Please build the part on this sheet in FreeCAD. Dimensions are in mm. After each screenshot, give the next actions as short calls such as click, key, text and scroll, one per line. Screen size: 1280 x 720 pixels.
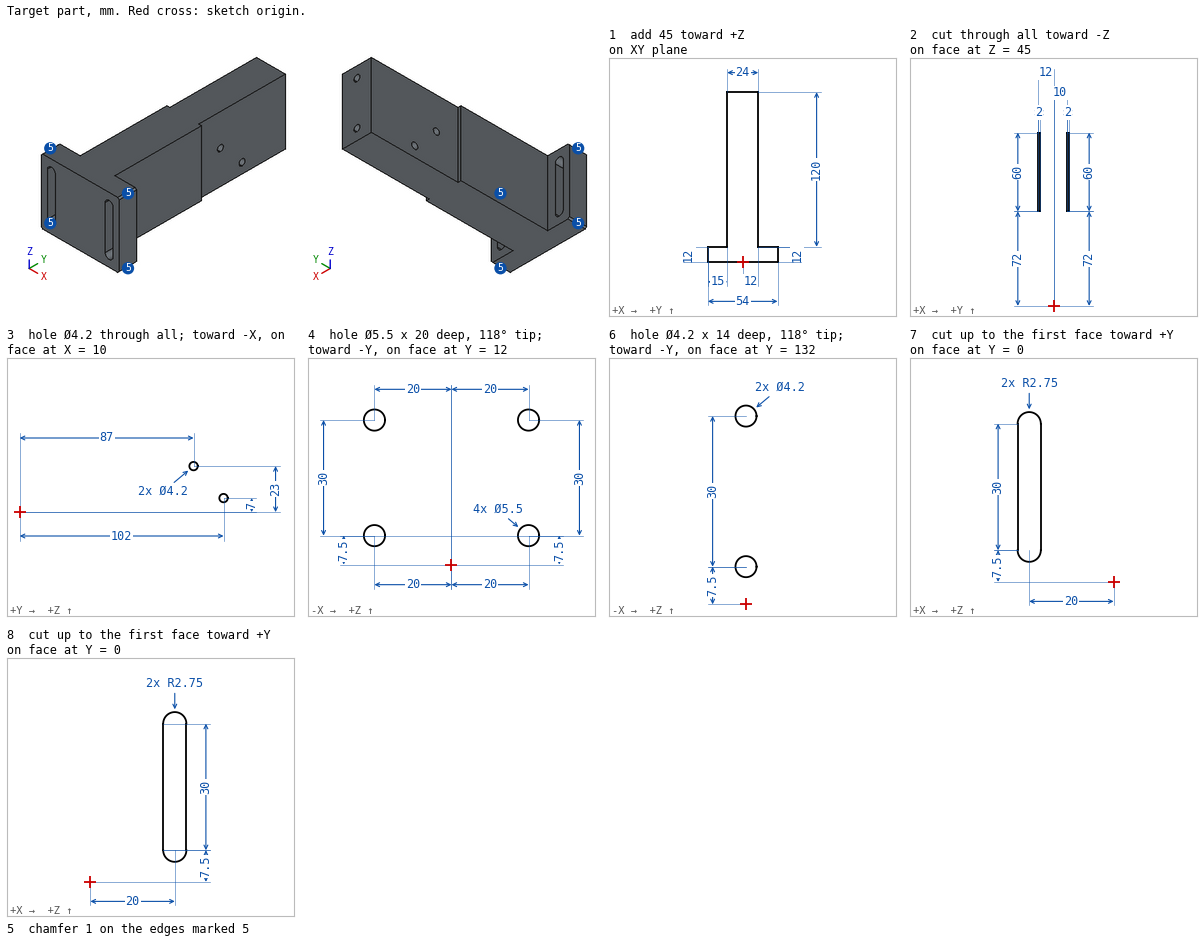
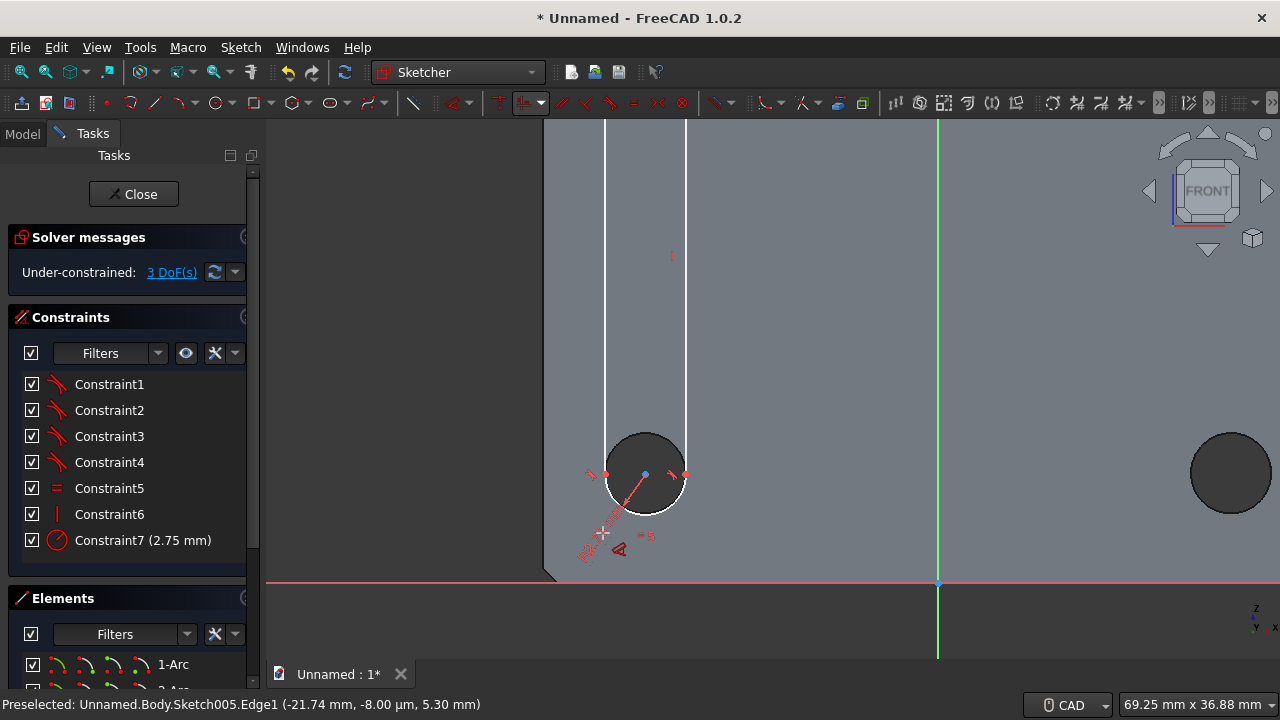
click(605, 343)
click(571, 311)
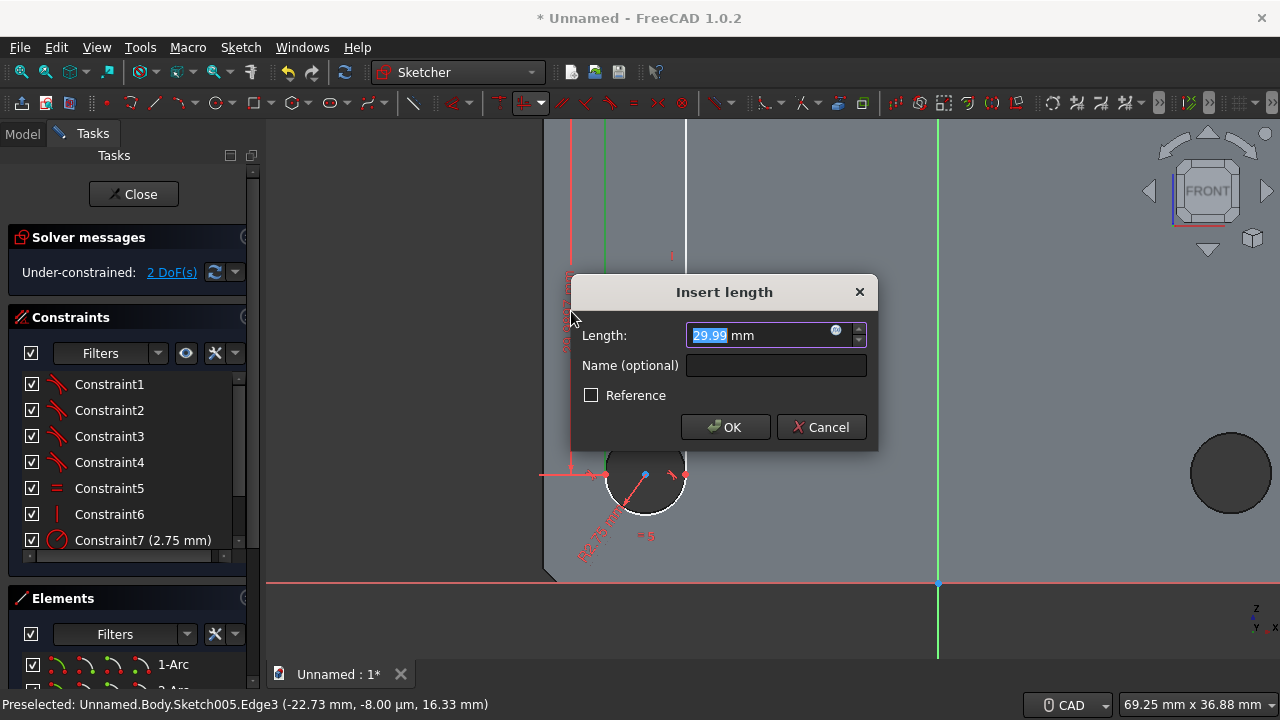
text(30)
key(Return)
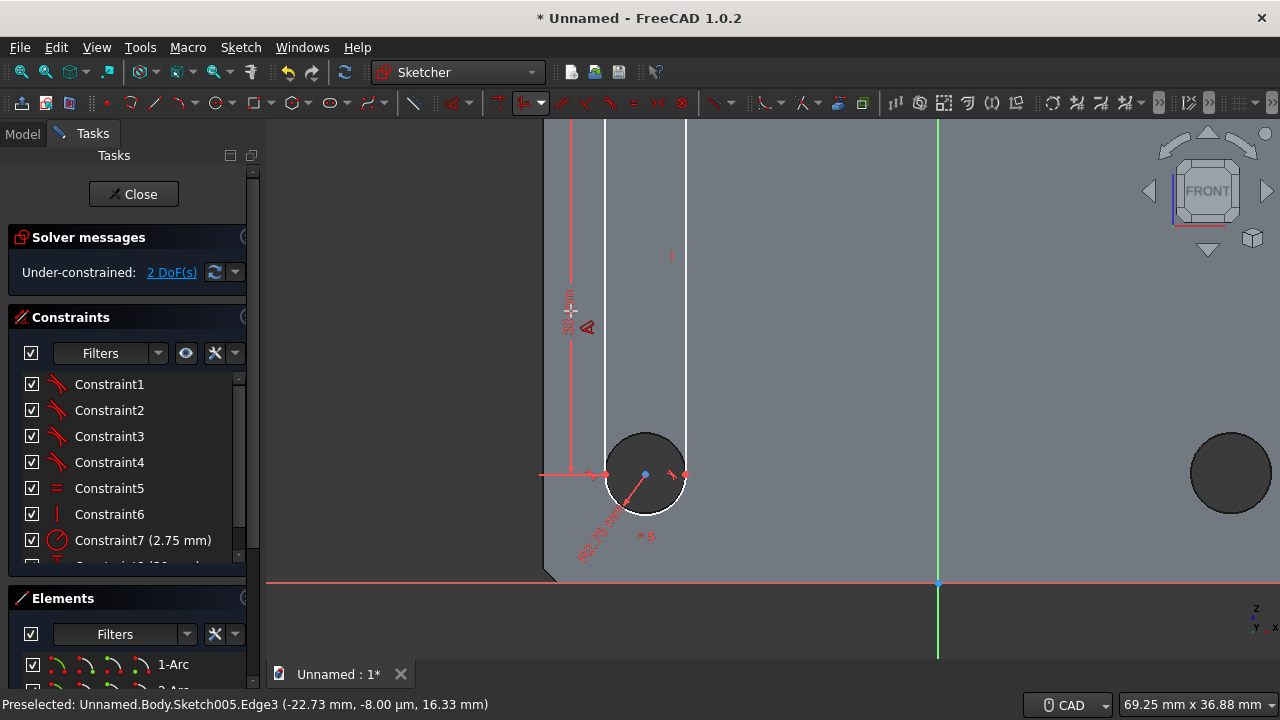
click(646, 475)
click(792, 617)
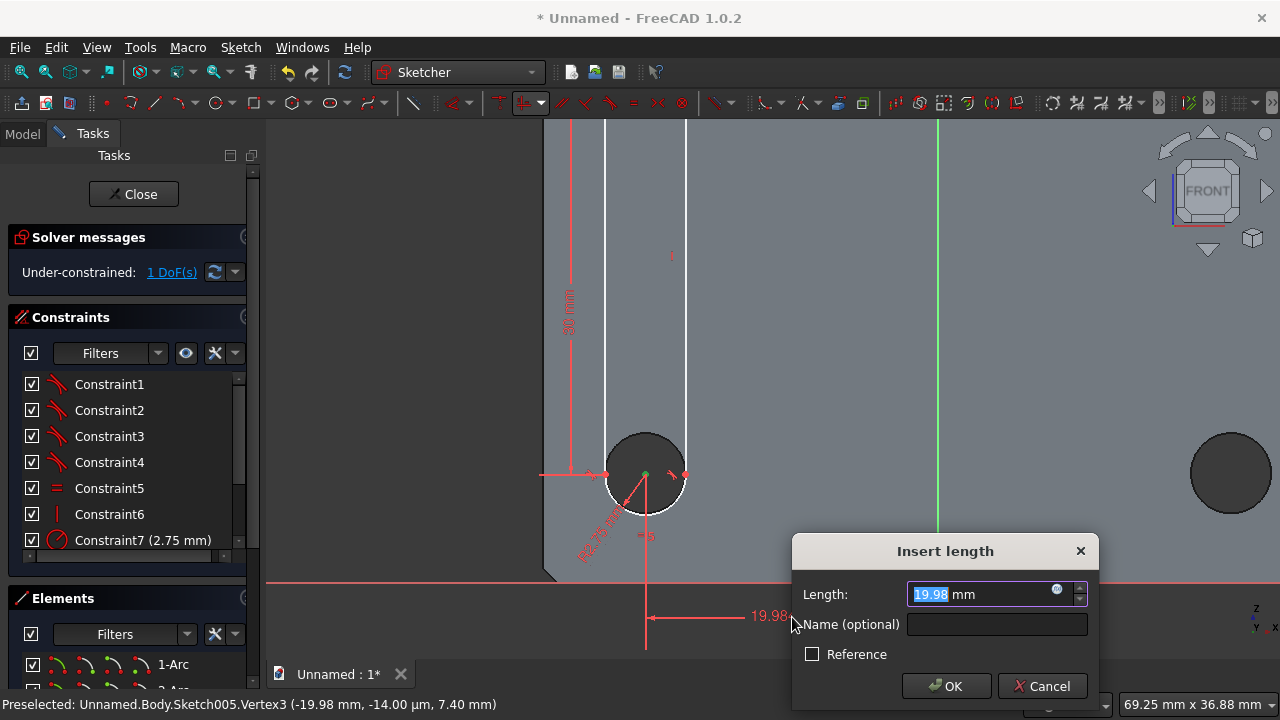
text(20)
key(Return)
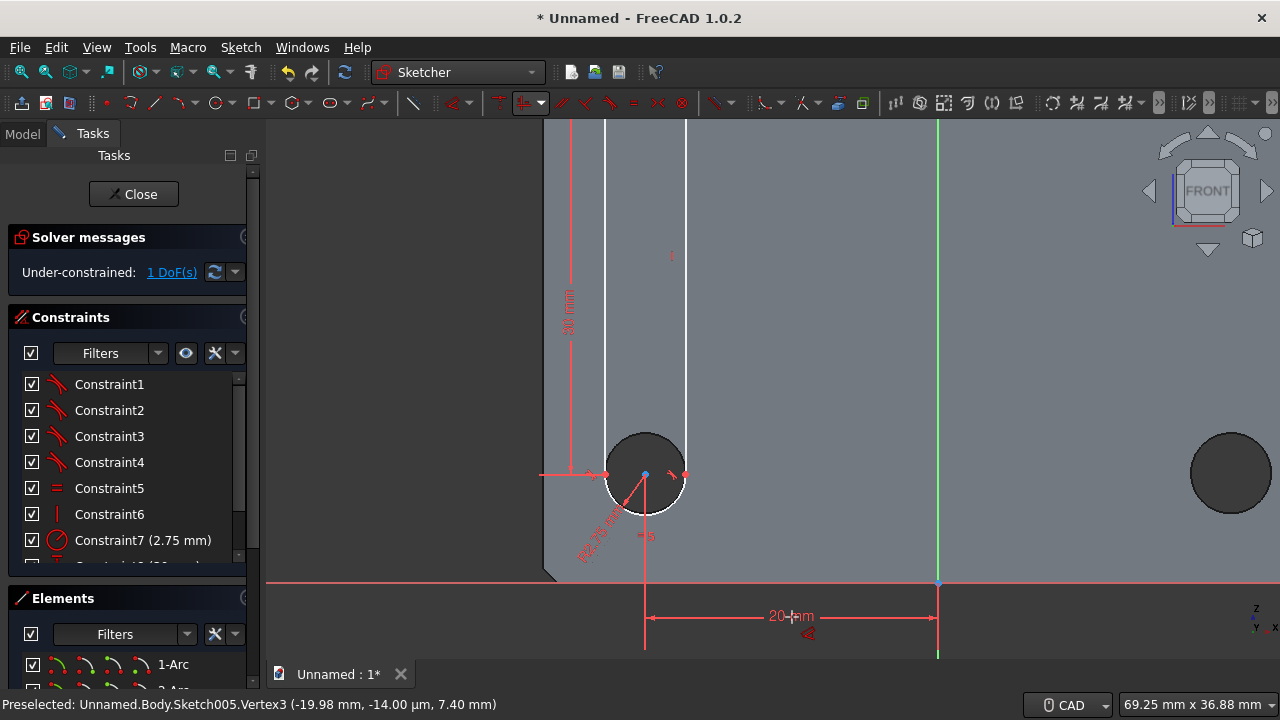
click(605, 475)
click(972, 529)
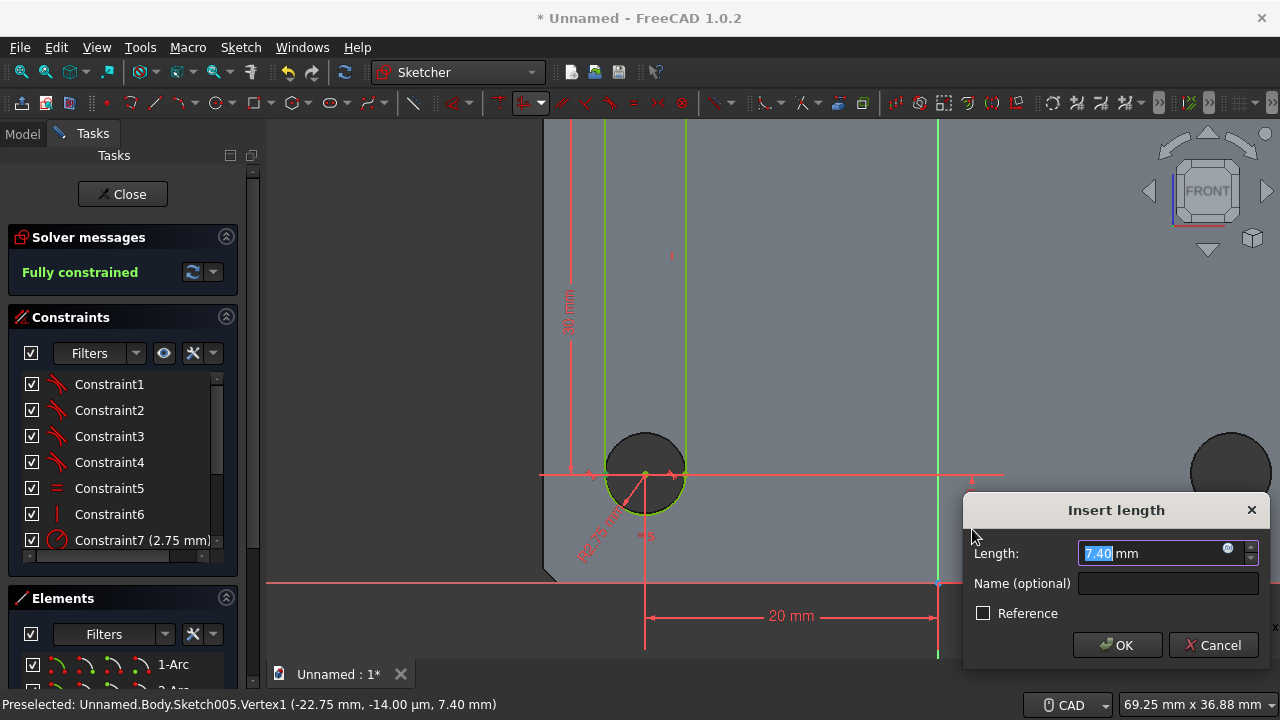
text(7.5)
key(Return)
key(Escape)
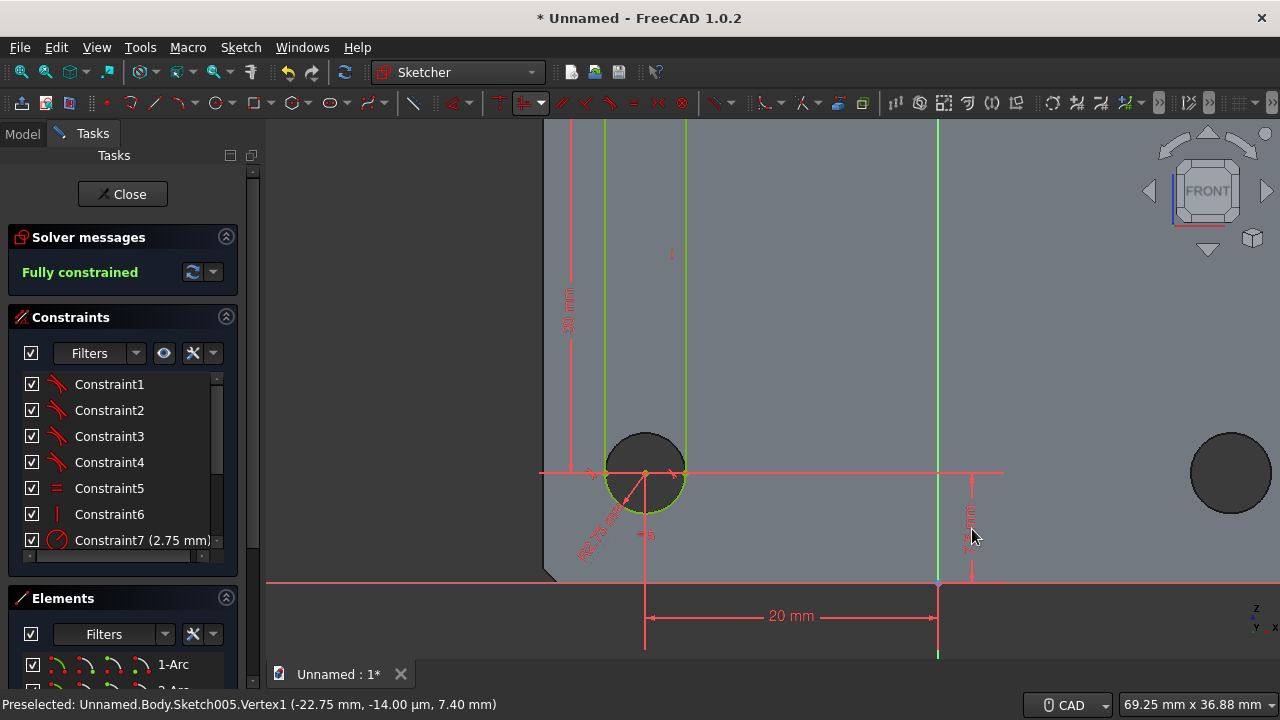
click(123, 194)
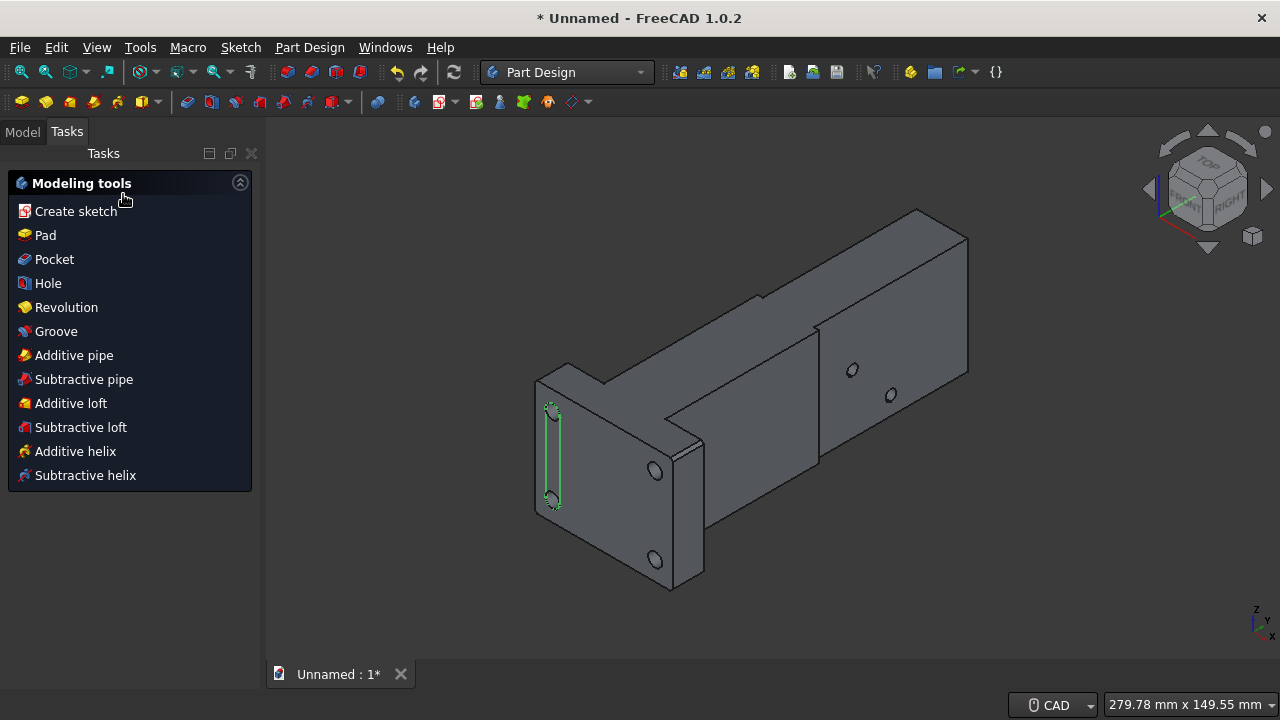
click(188, 102)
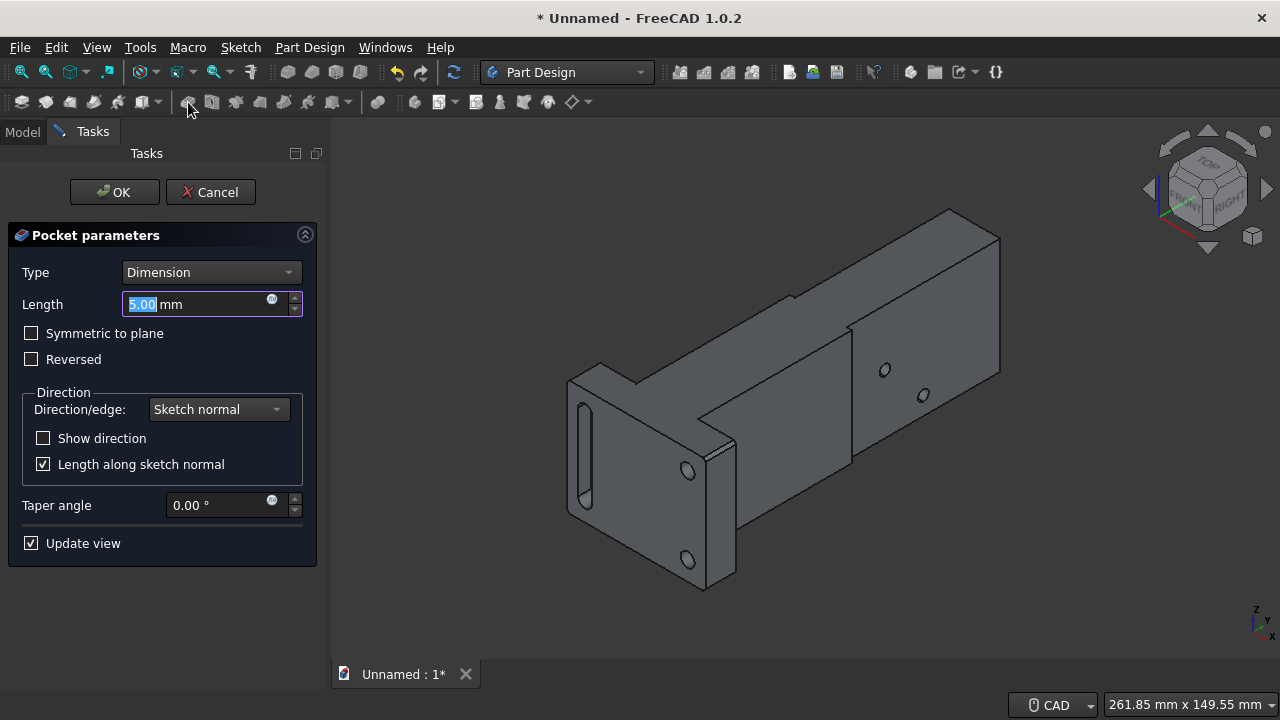
click(212, 272)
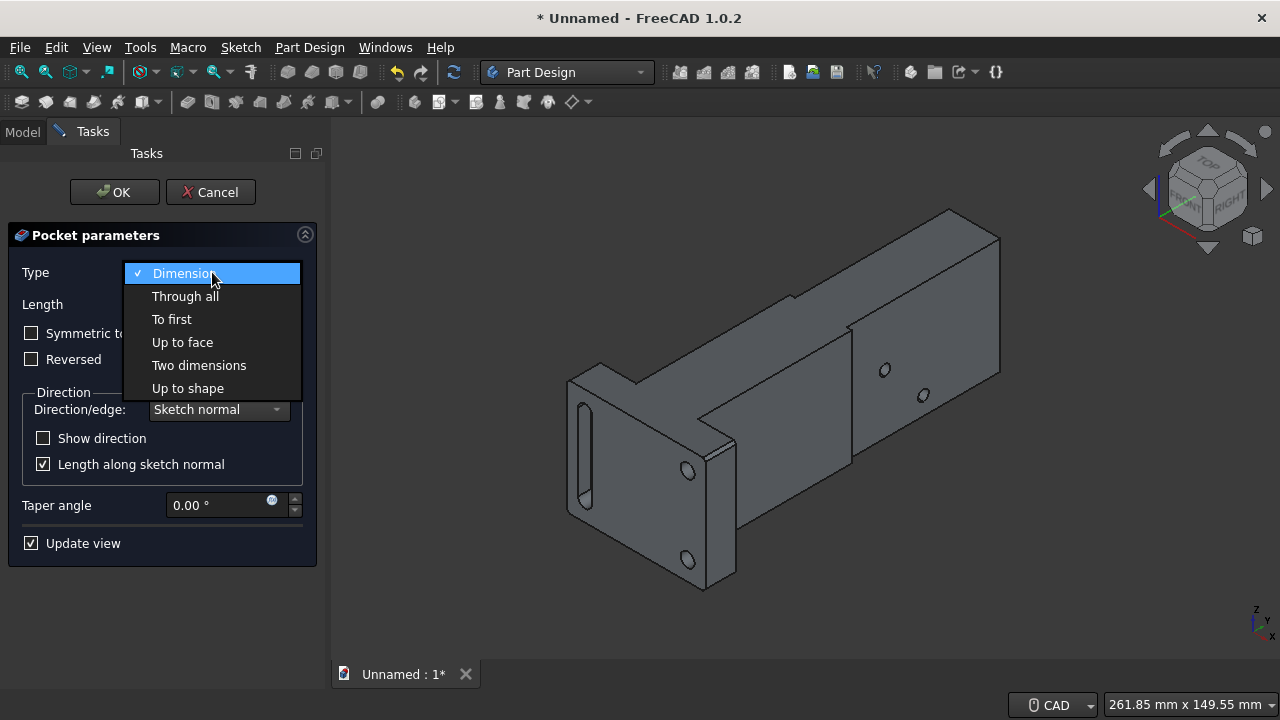
click(212, 320)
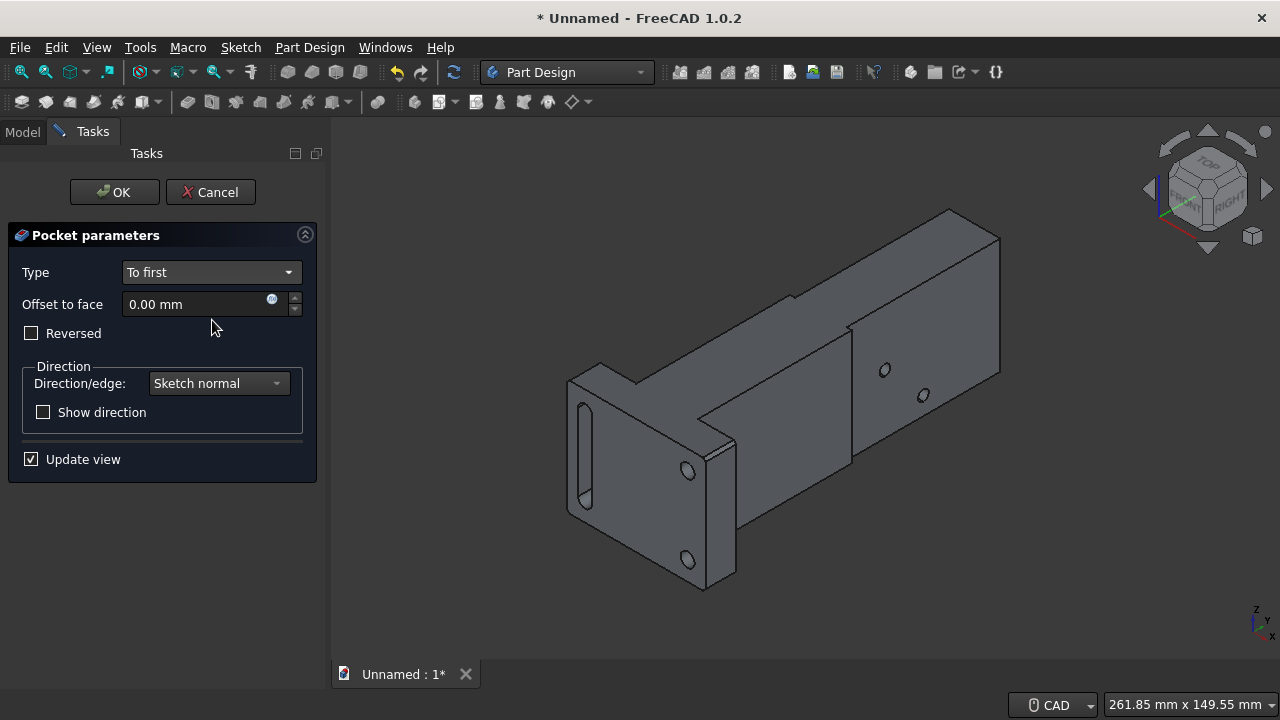
click(115, 192)